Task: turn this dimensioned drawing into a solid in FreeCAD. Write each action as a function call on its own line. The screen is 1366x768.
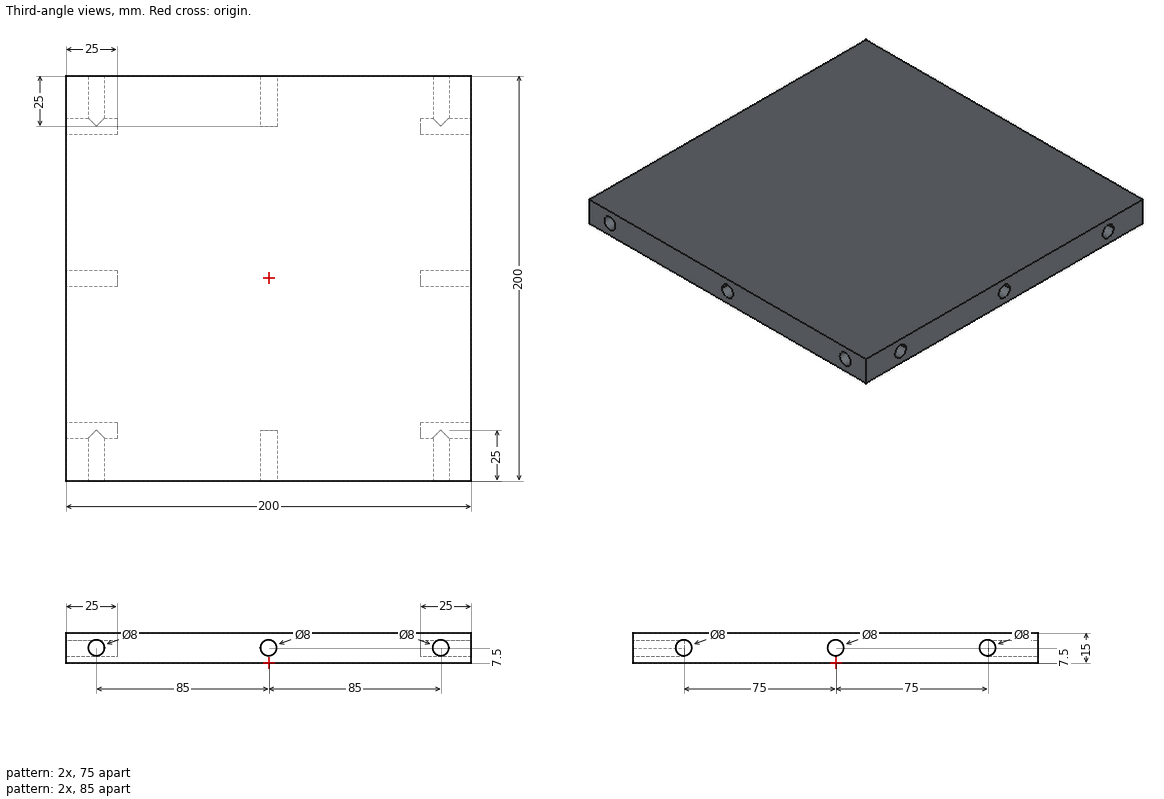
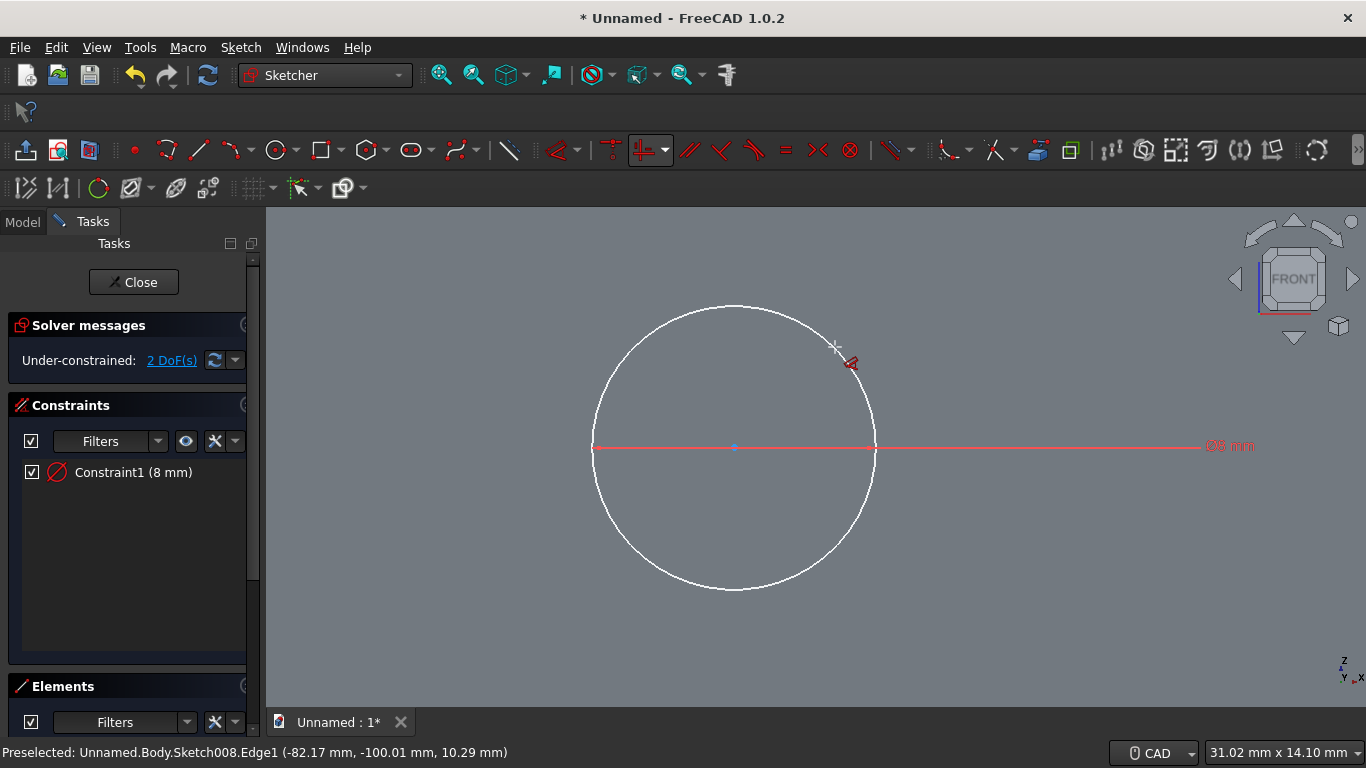
click(734, 448)
click(968, 414)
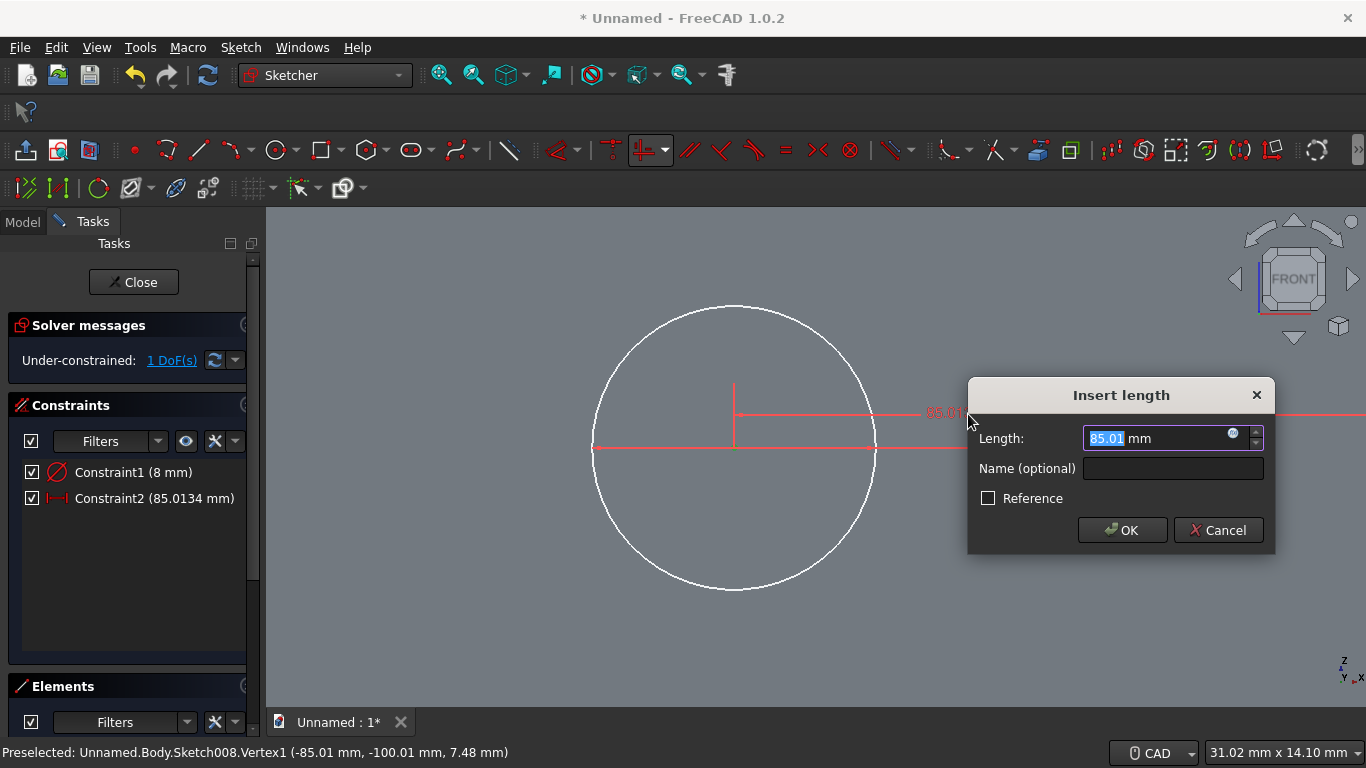
text(85)
key(Return)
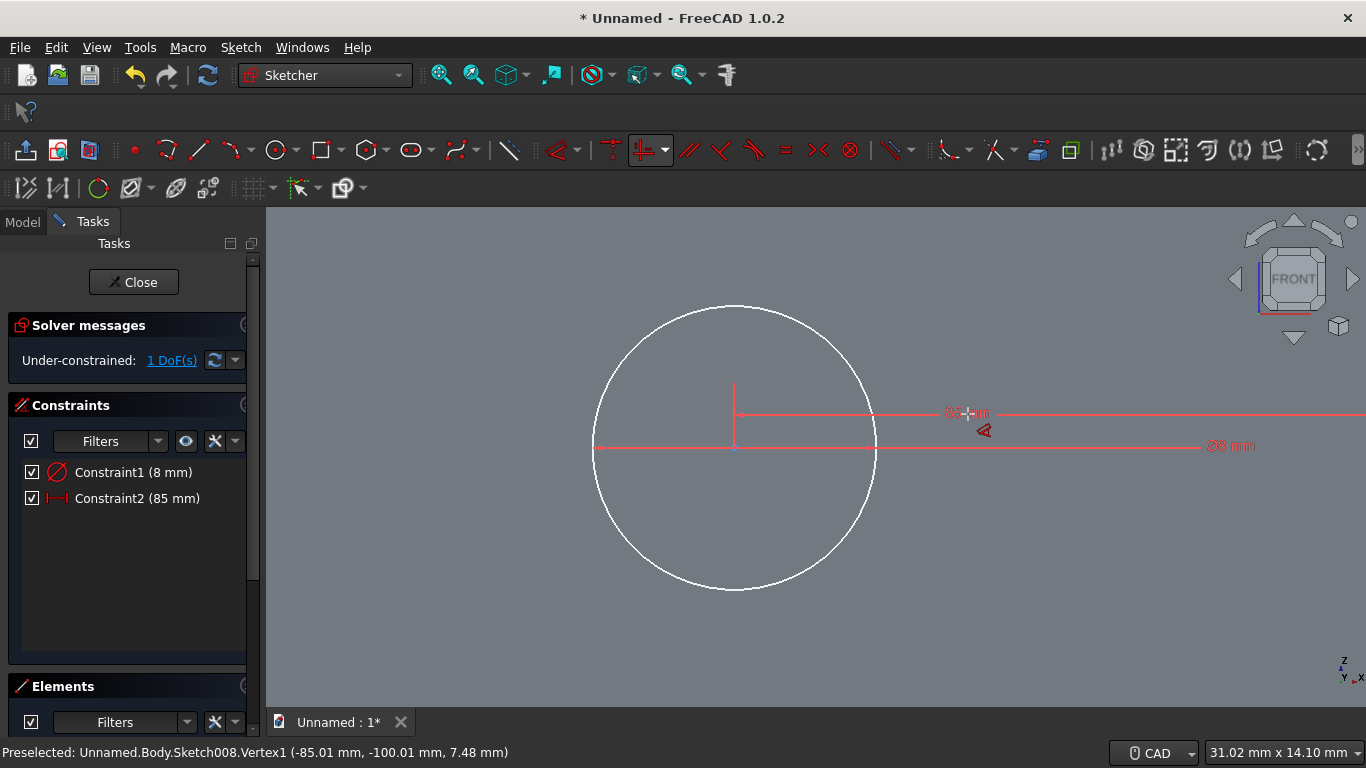
click(734, 448)
click(700, 563)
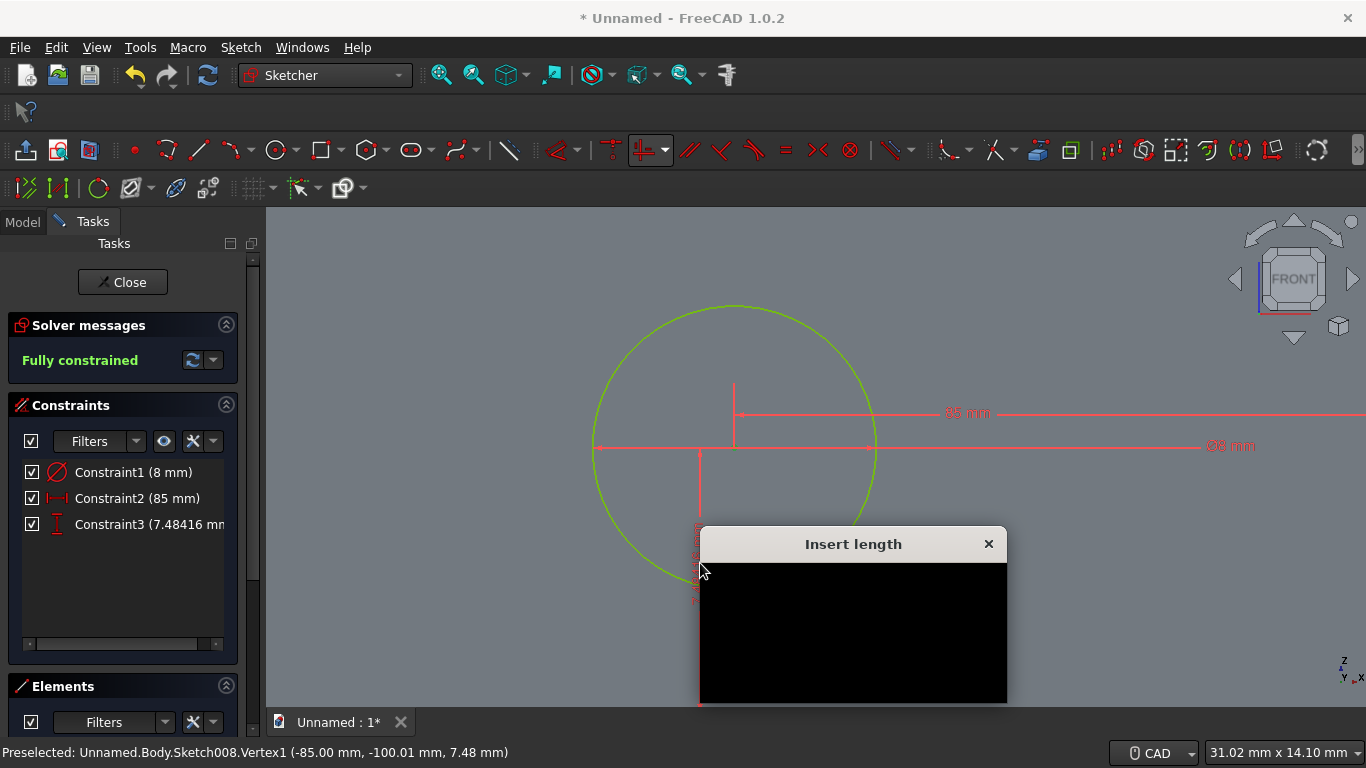
text(7.5)
key(Return)
key(Escape)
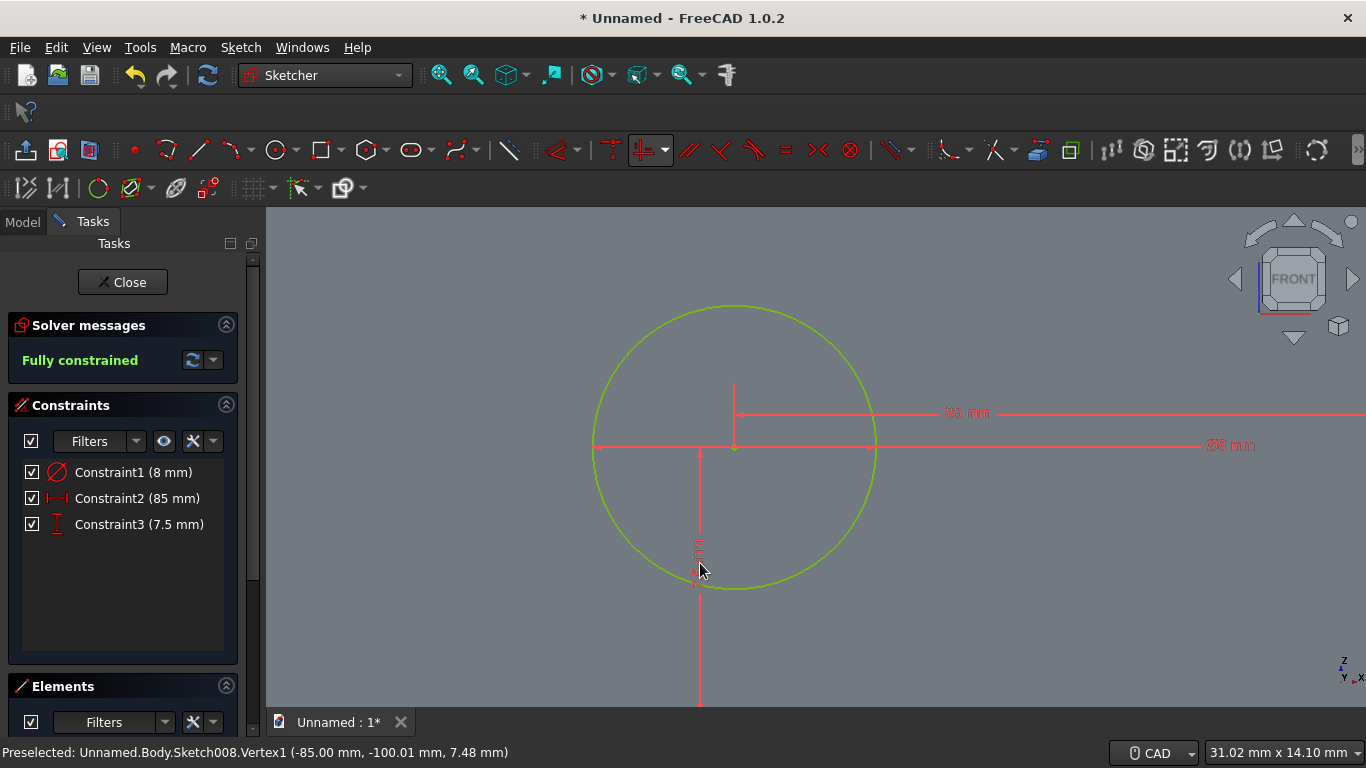
click(123, 282)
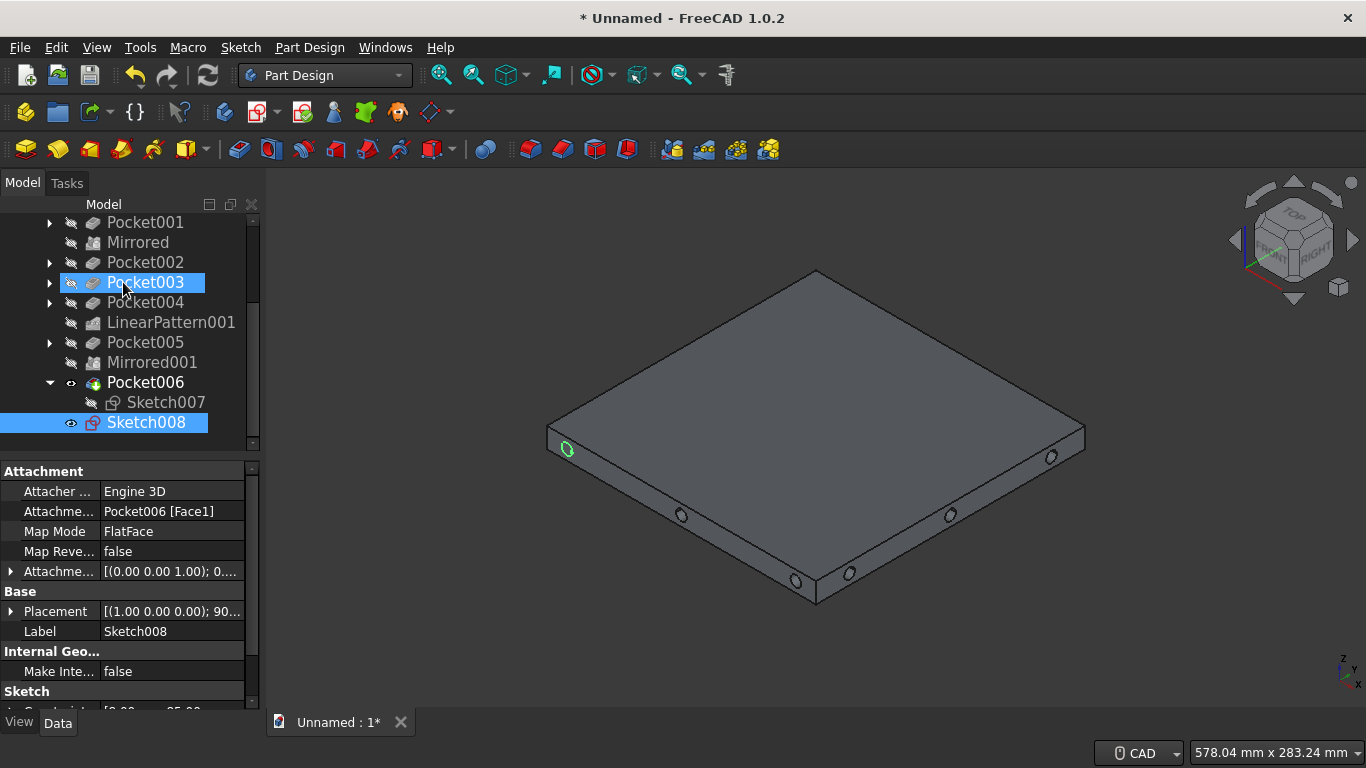
click(240, 150)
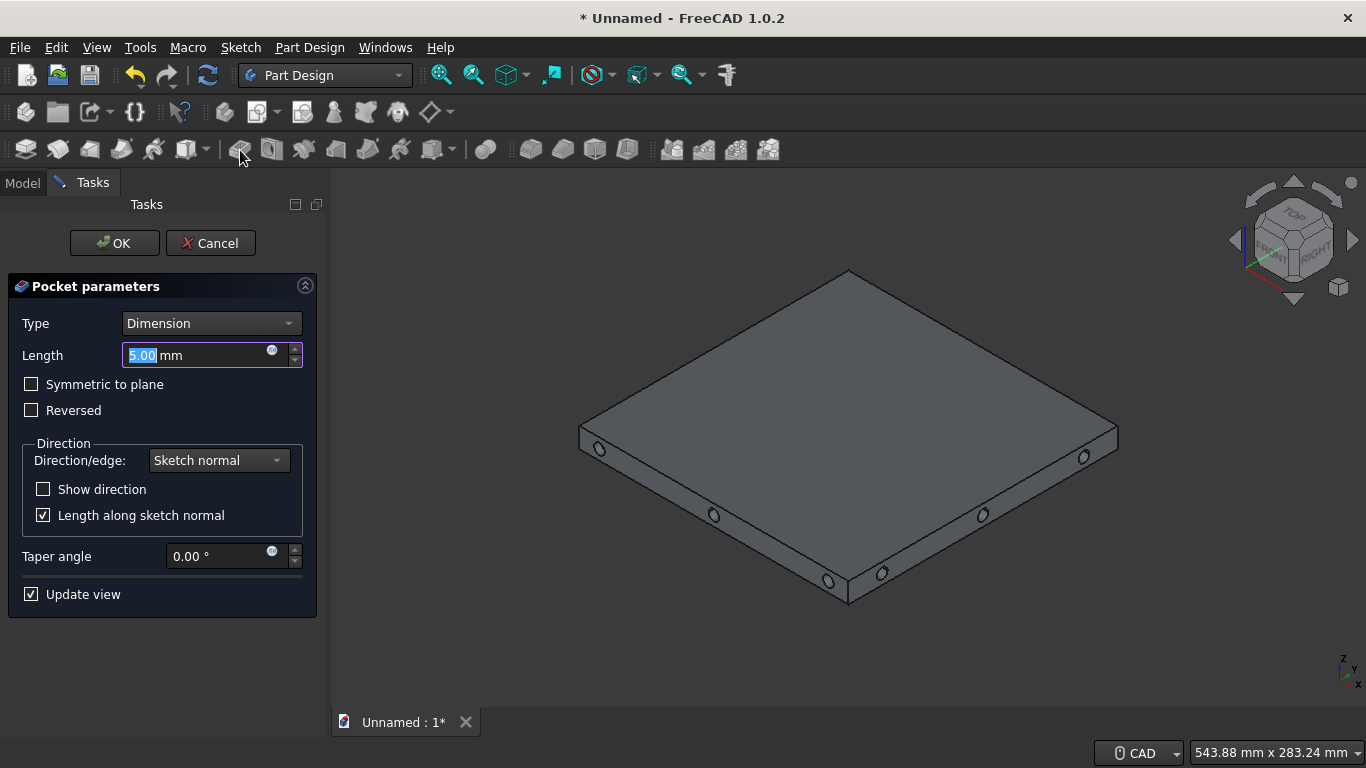
text(25)
key(Tab)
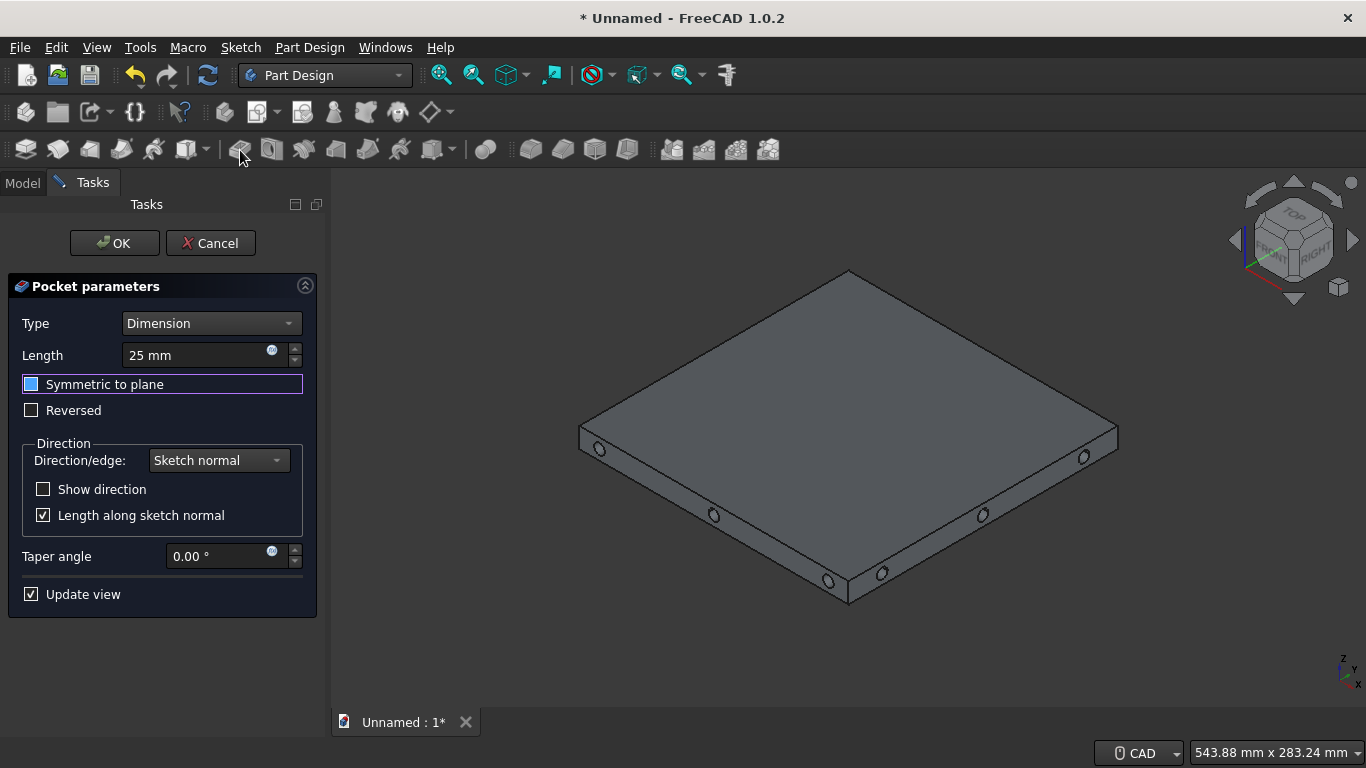
click(115, 243)